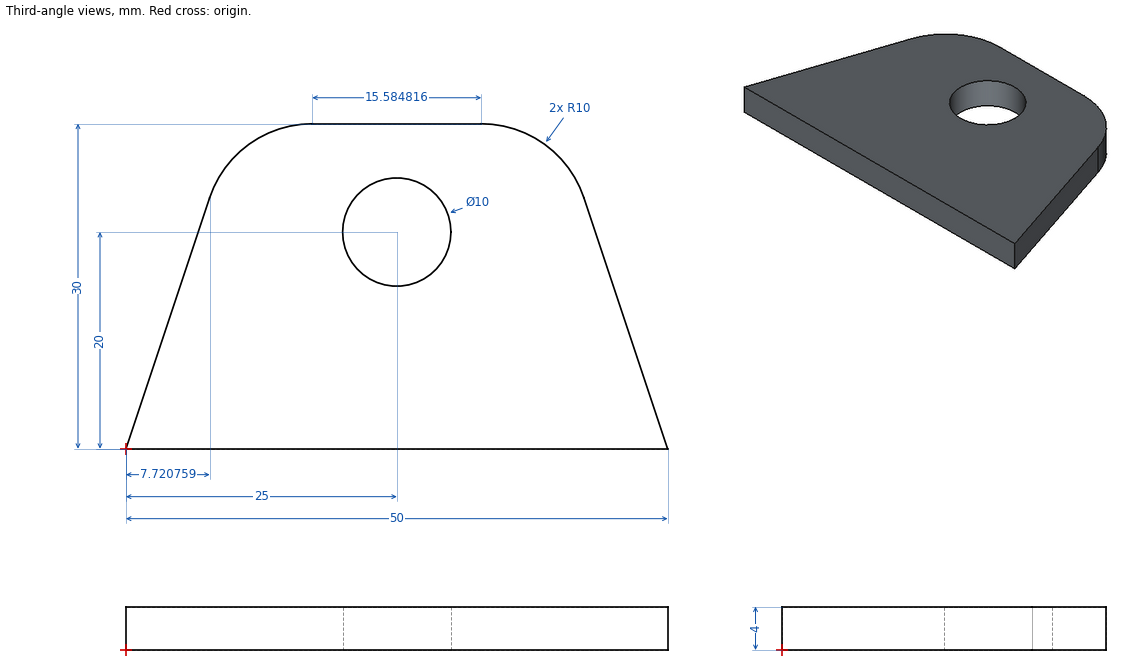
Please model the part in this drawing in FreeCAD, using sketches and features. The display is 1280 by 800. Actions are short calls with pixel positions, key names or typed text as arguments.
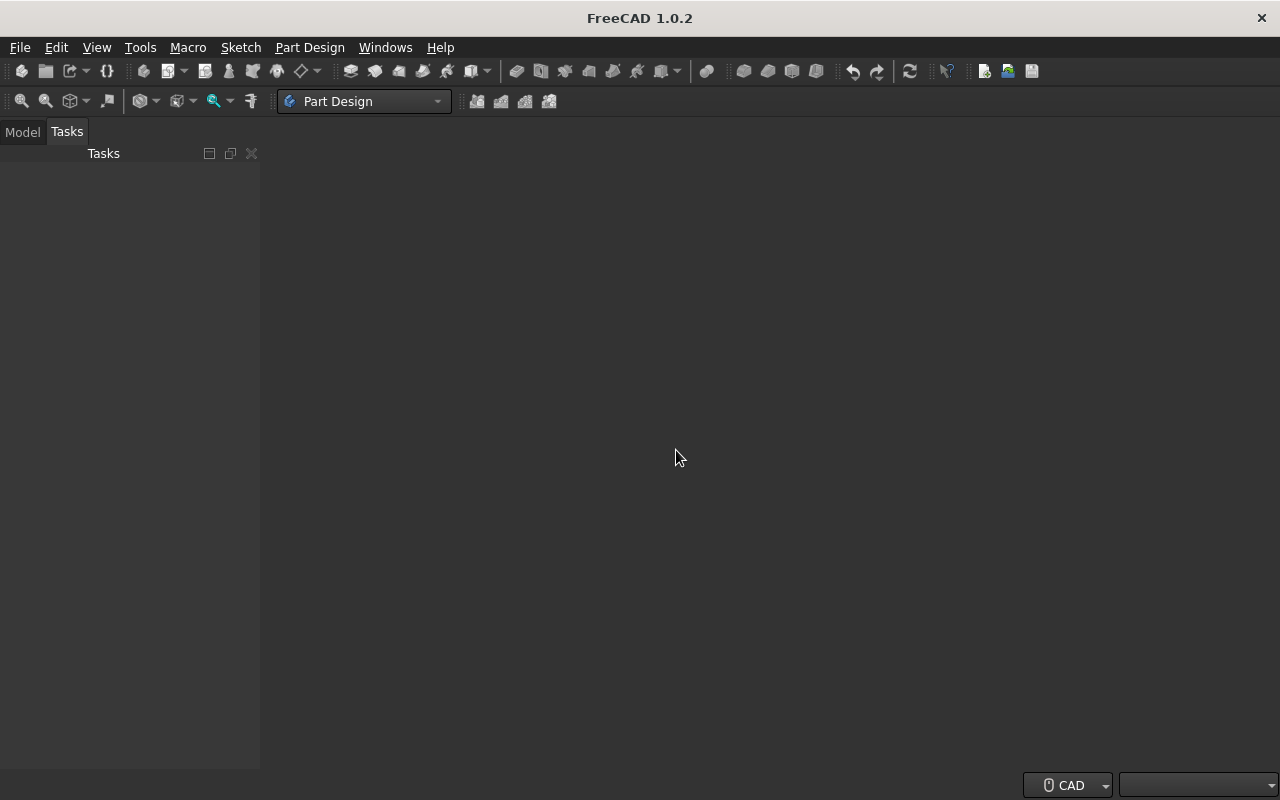
click(984, 72)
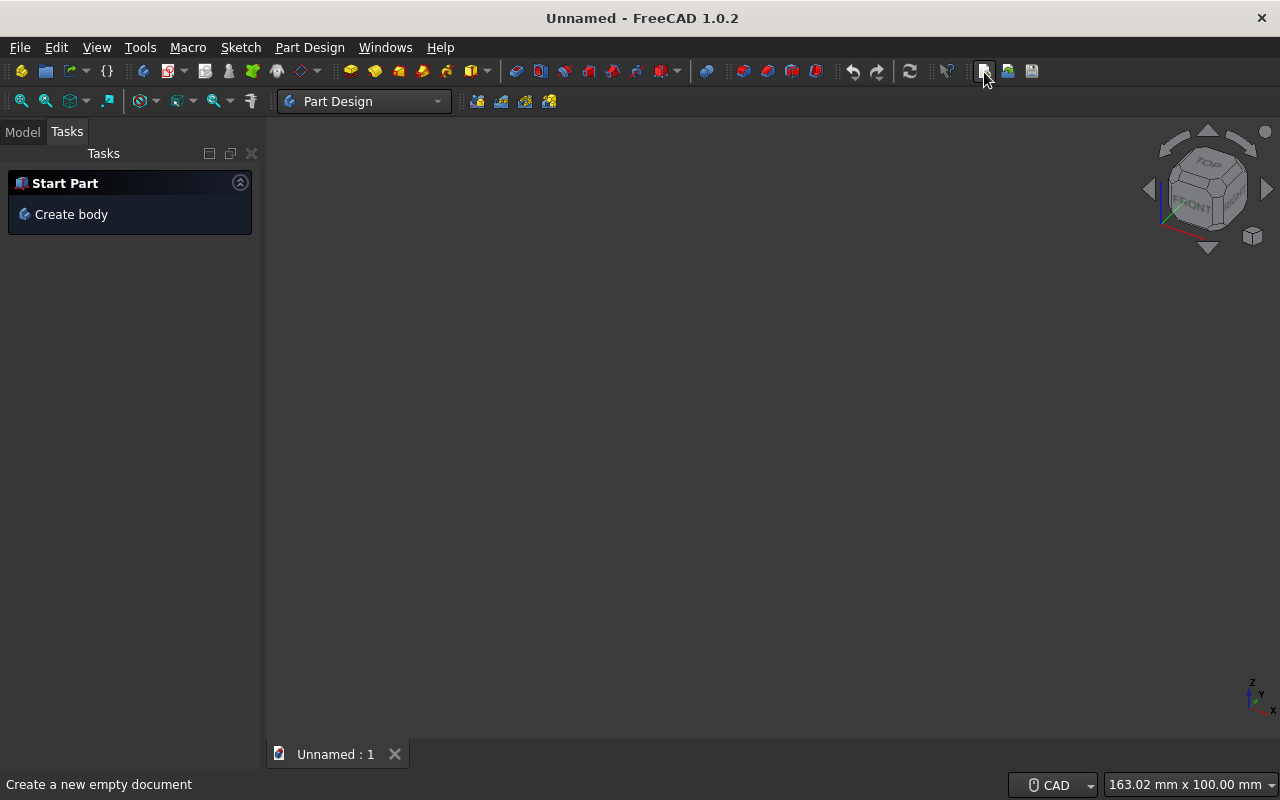
click(168, 72)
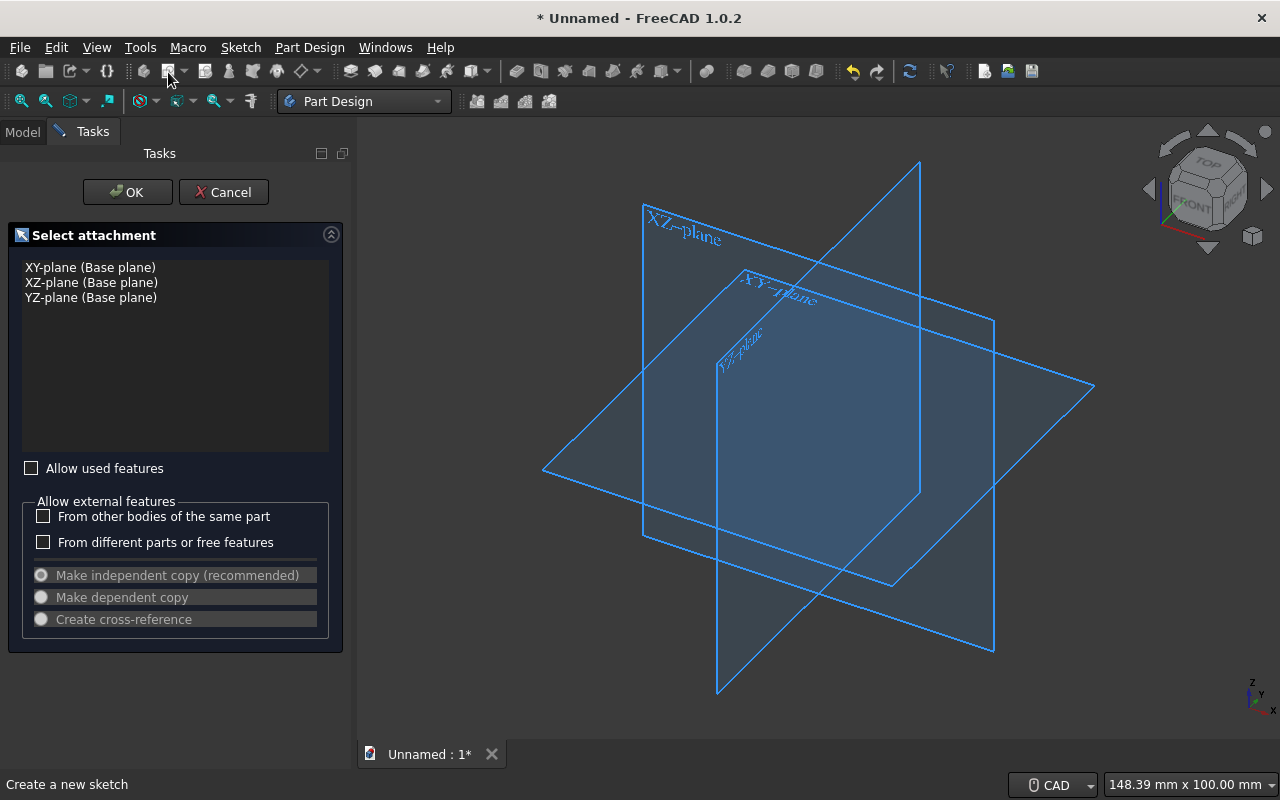
click(82, 268)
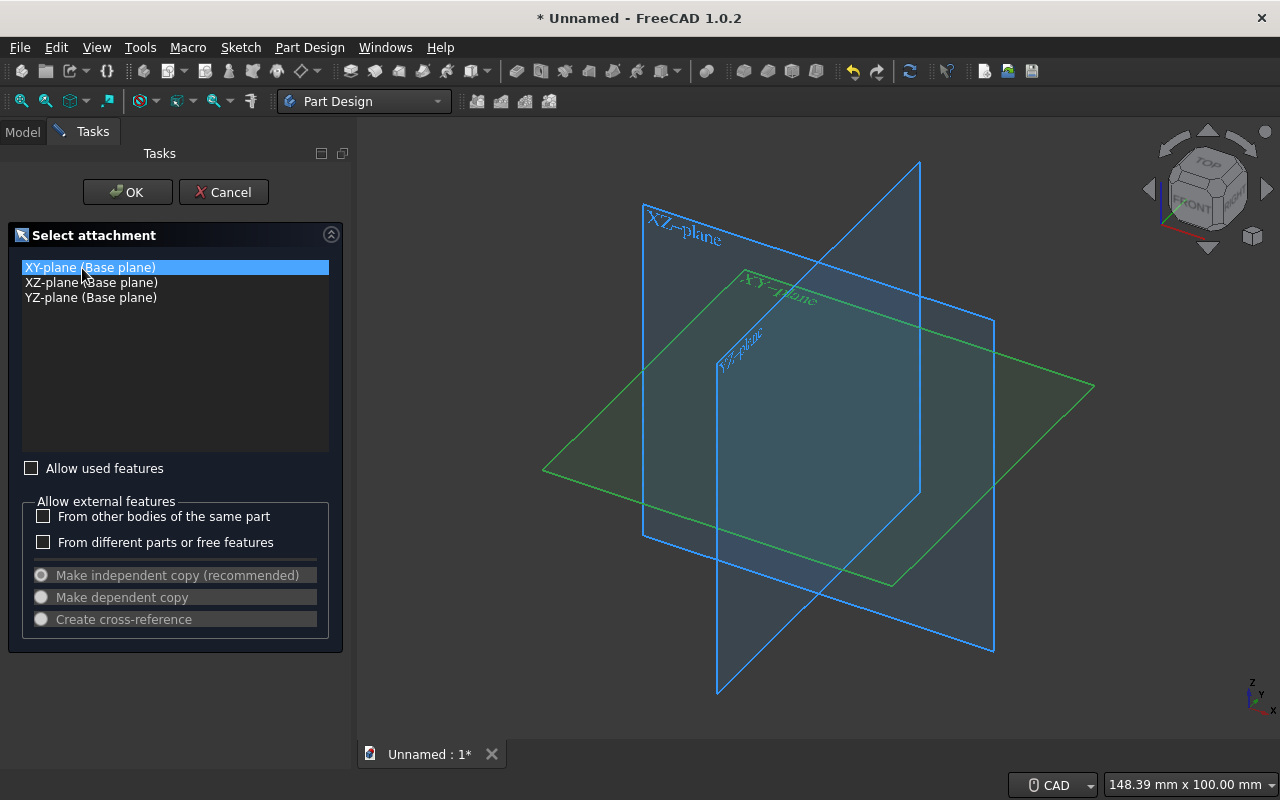
click(128, 192)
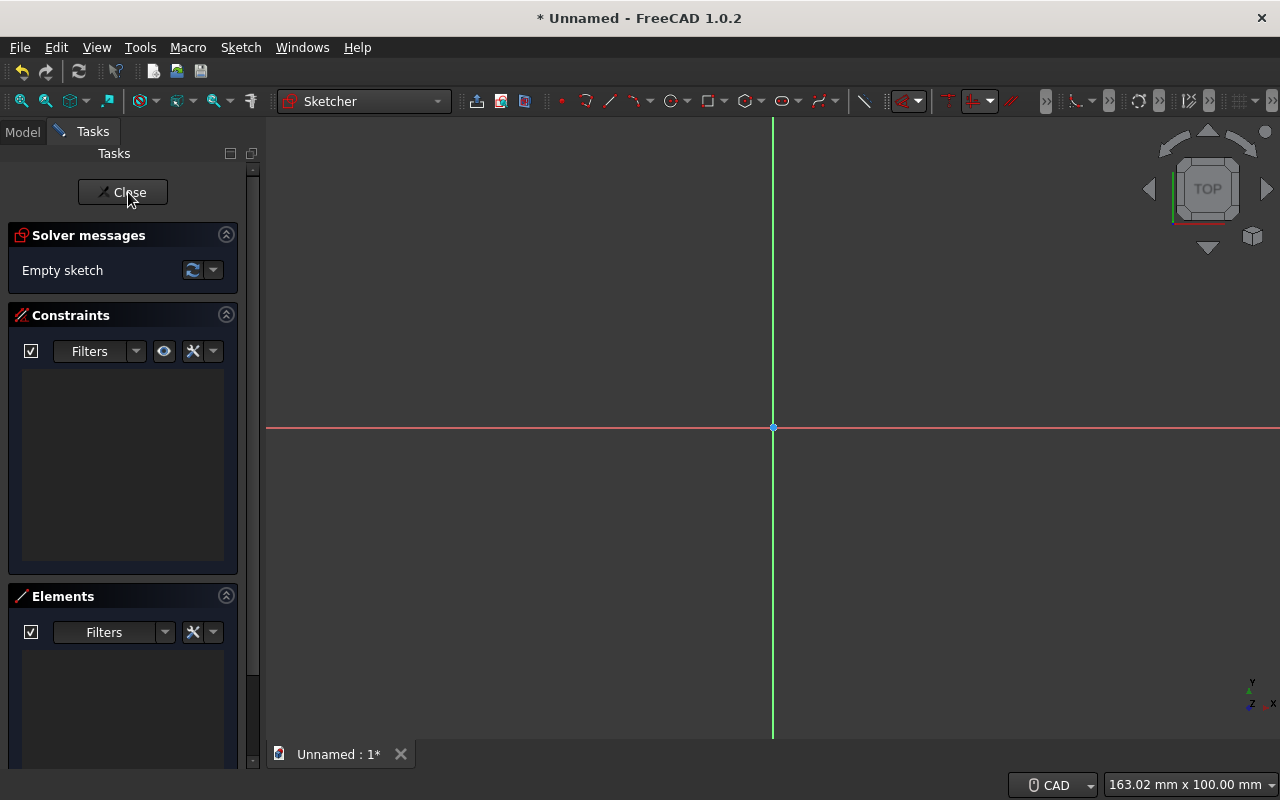
scroll(1115, 221, up, 3)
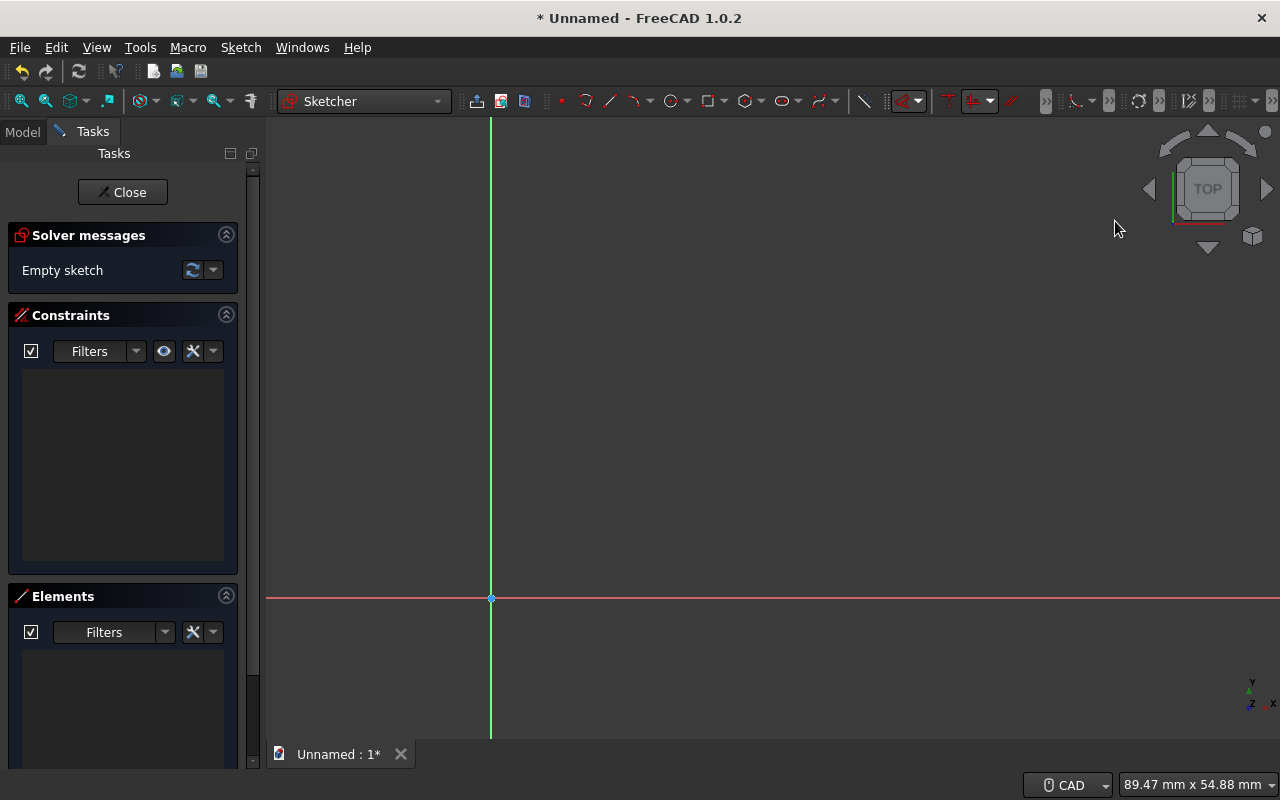
click(610, 102)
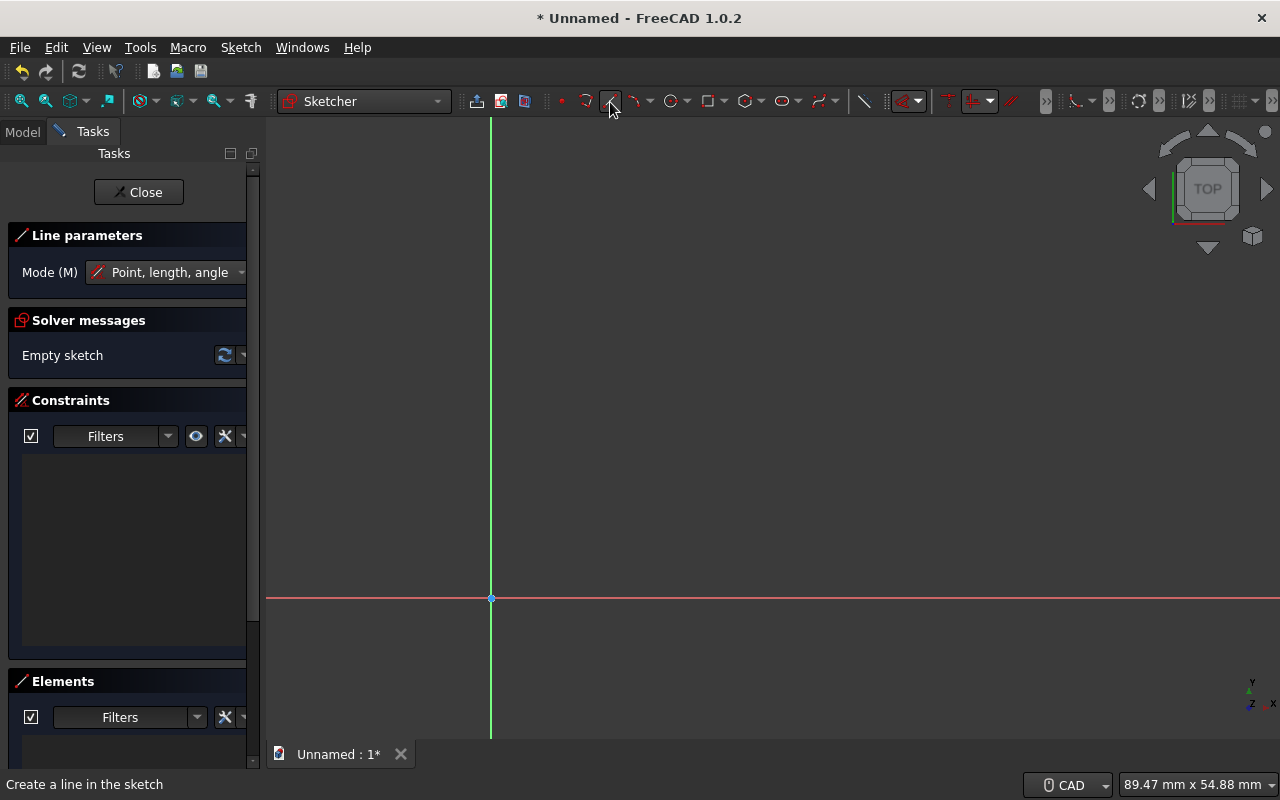
click(863, 258)
click(686, 258)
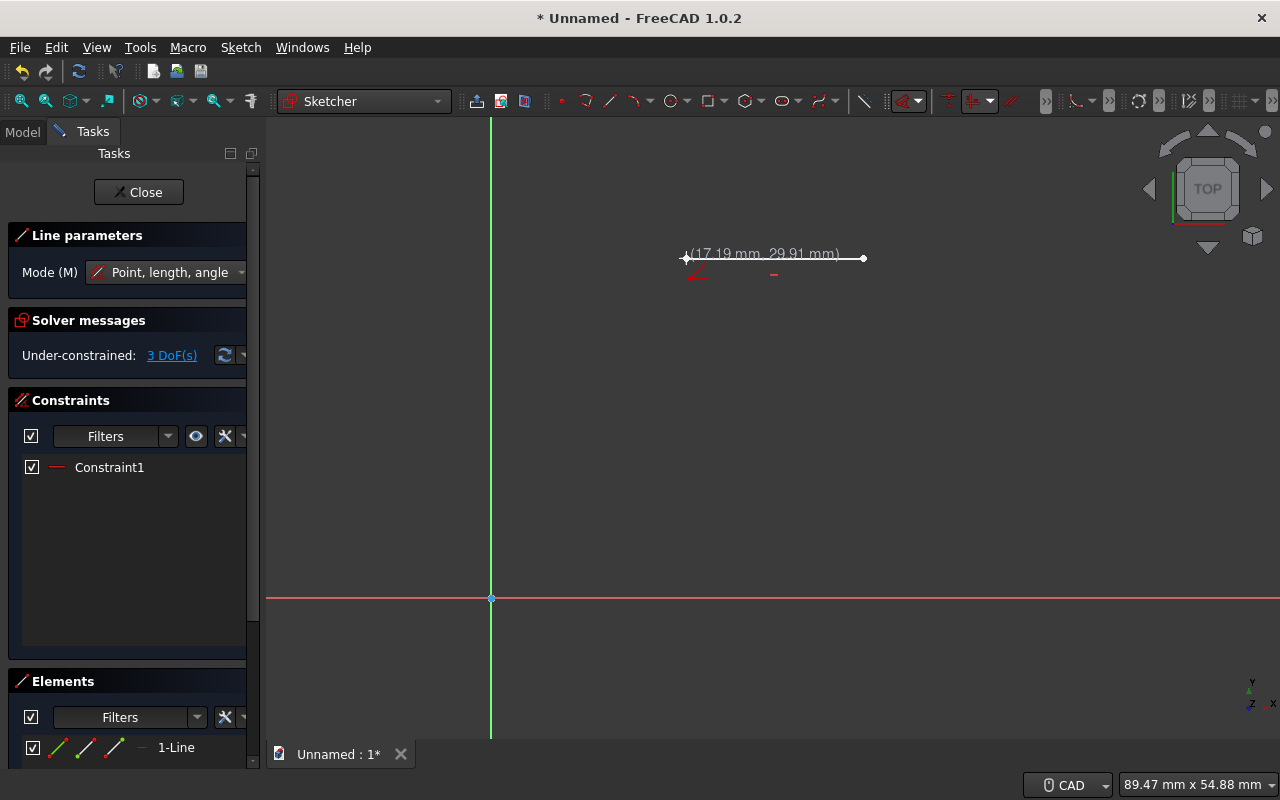
key(g)
key(m)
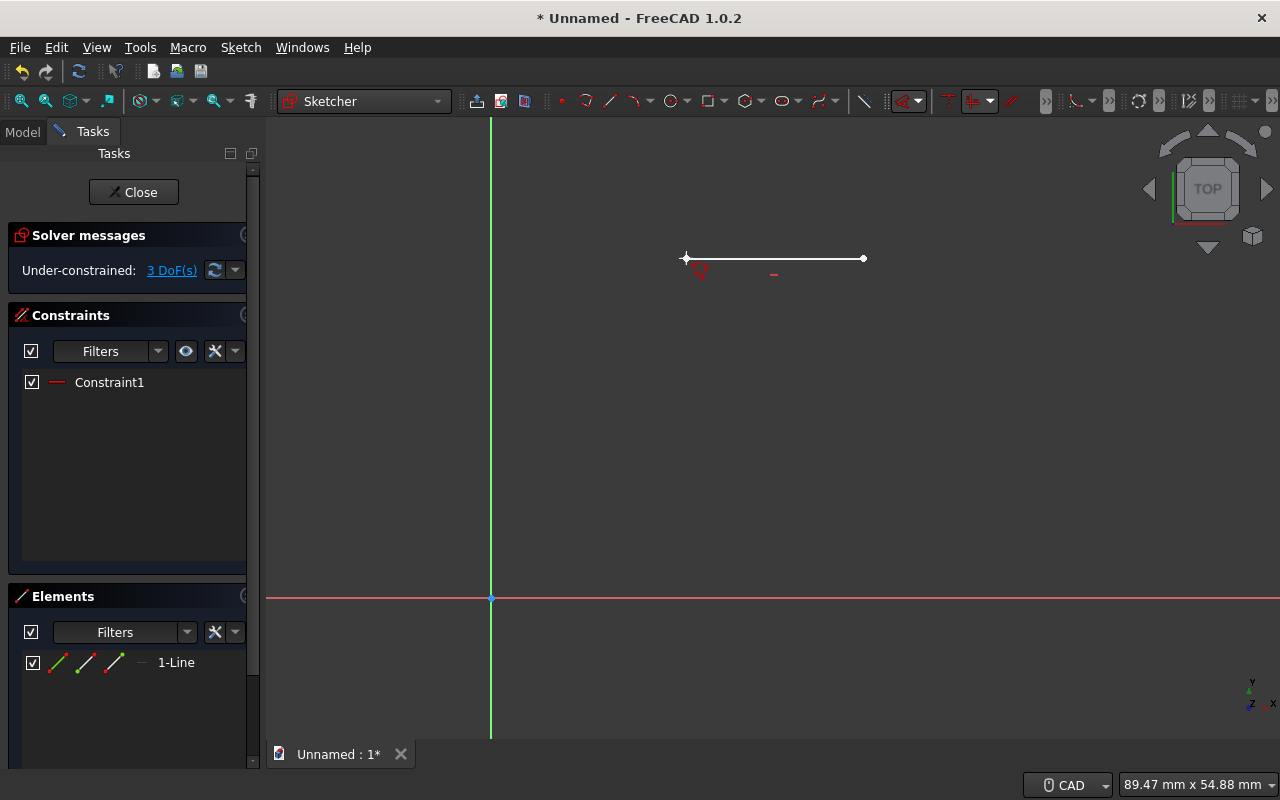
click(579, 336)
click(491, 598)
click(1058, 589)
click(970, 336)
right_click(970, 336)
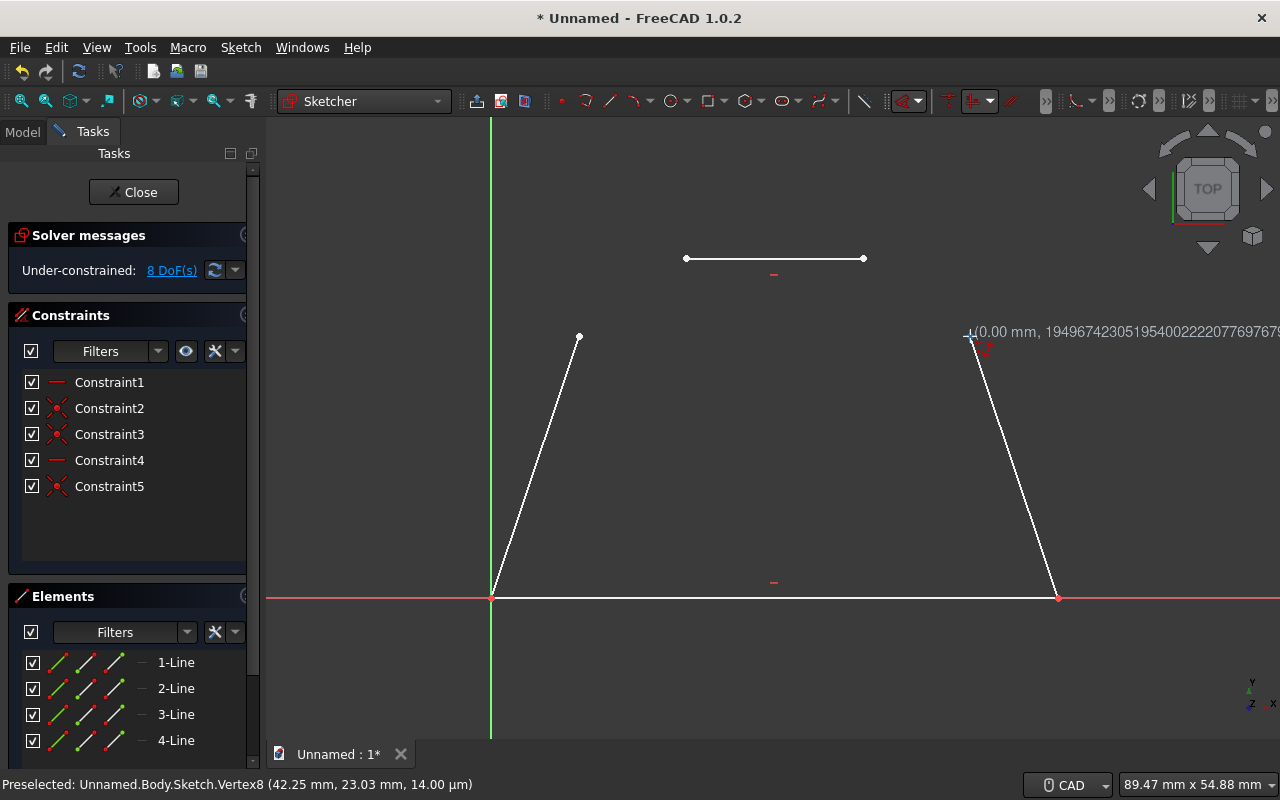
click(634, 102)